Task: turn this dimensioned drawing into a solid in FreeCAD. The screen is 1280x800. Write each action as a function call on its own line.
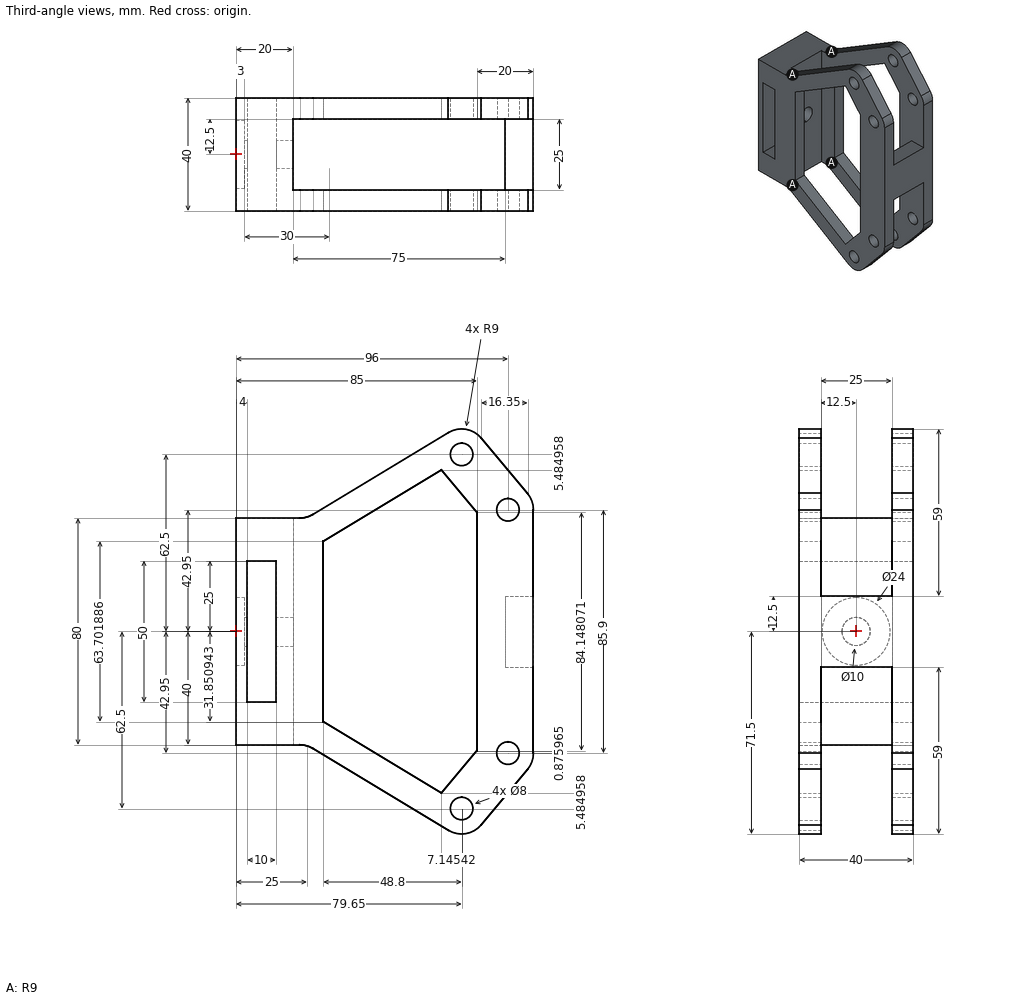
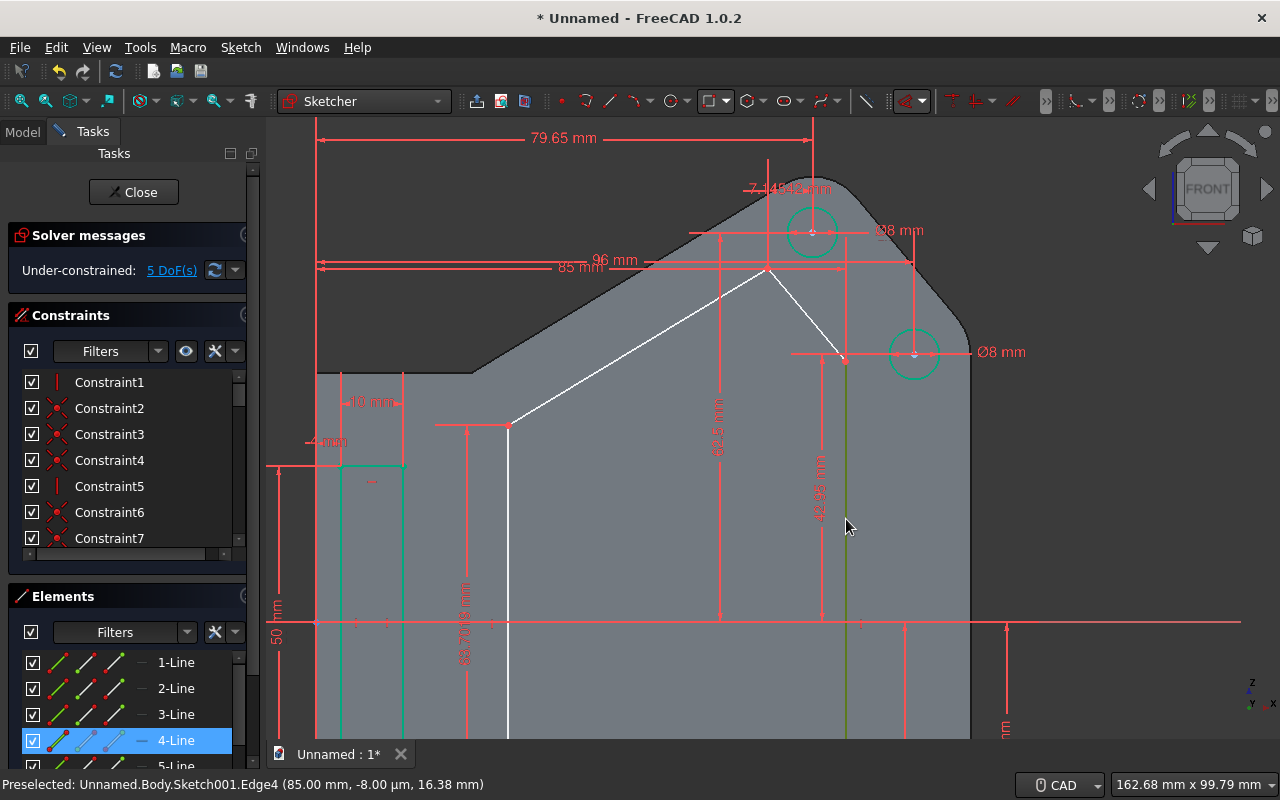
key(i)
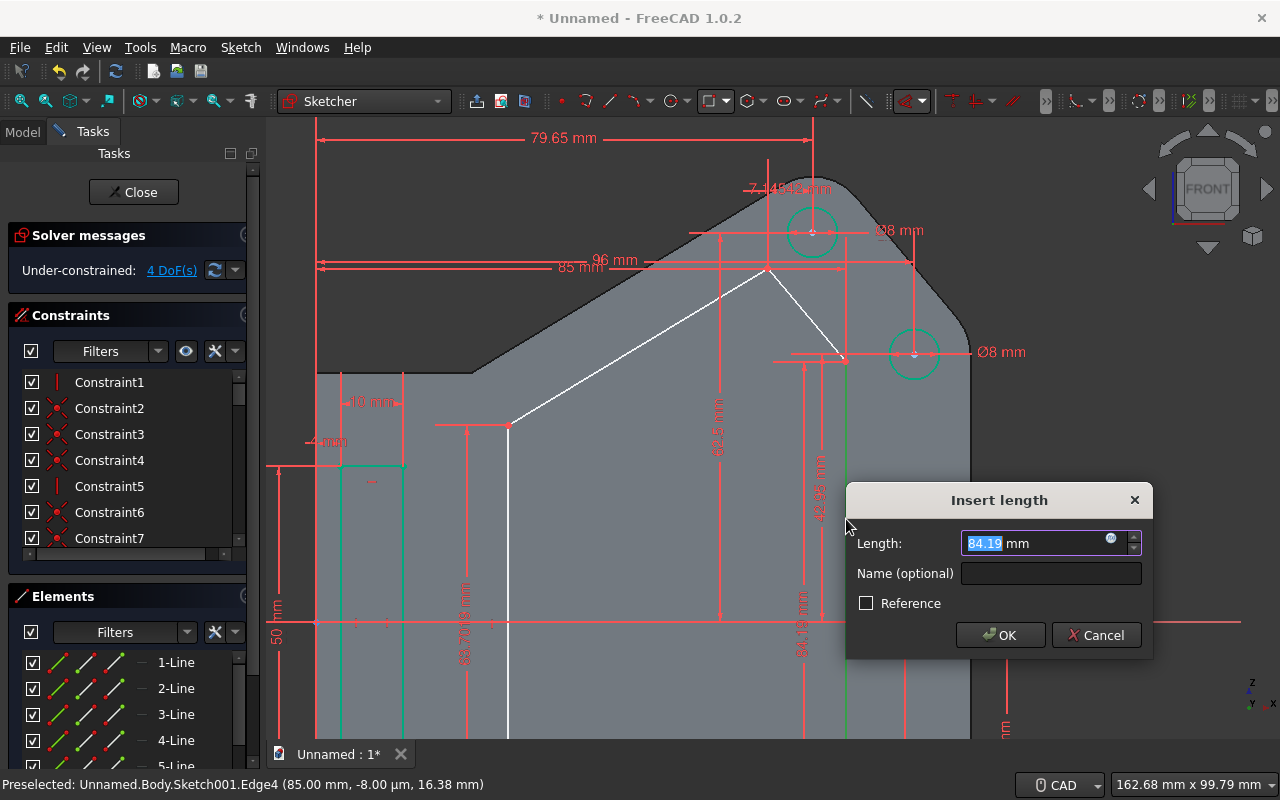
text(84.148071)
key(Return)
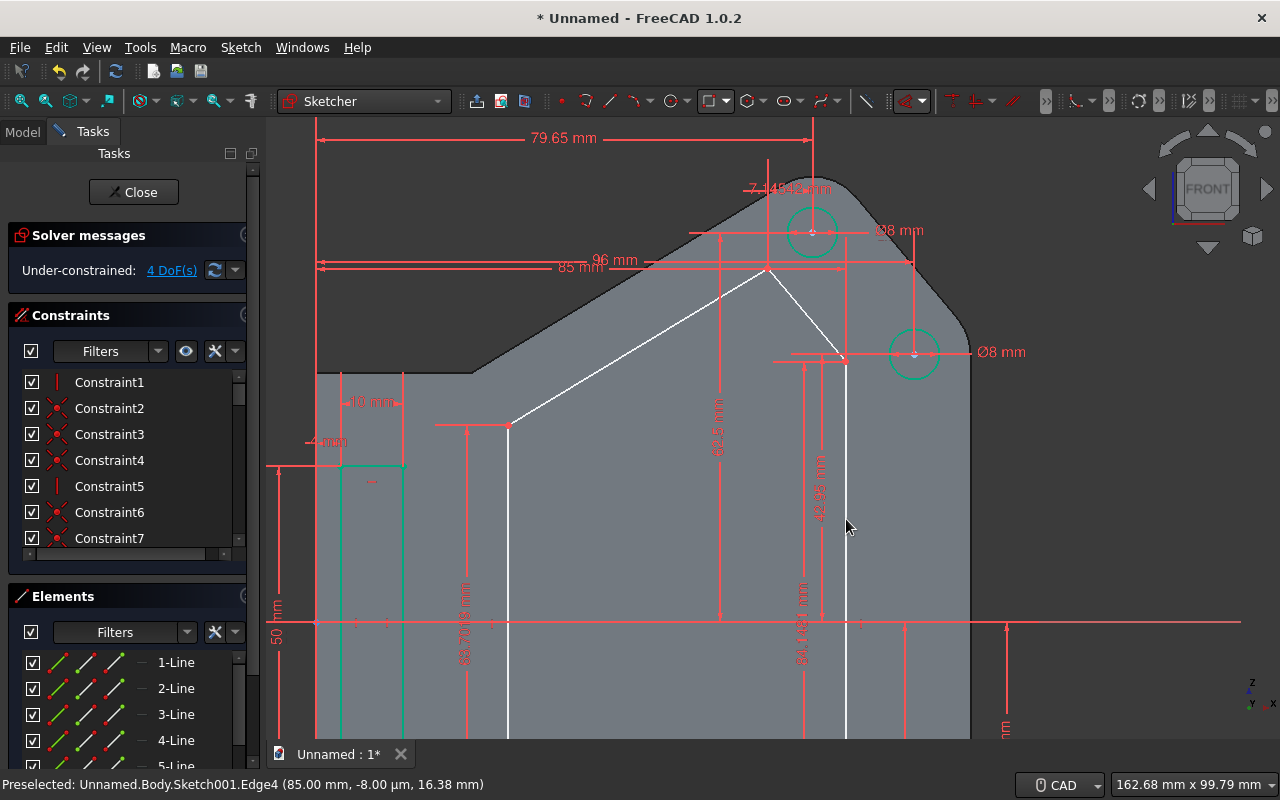
scroll(767, 270, down, 4)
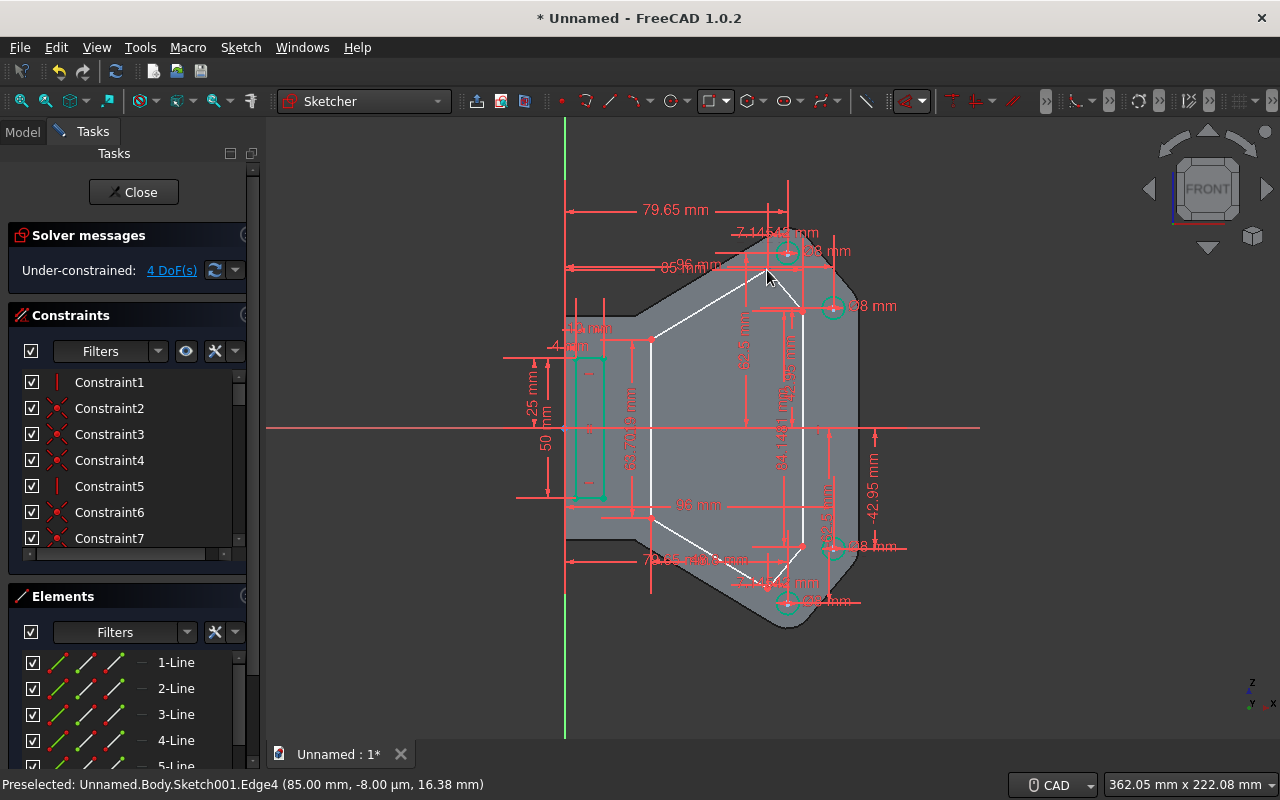
scroll(768, 589, up, 5)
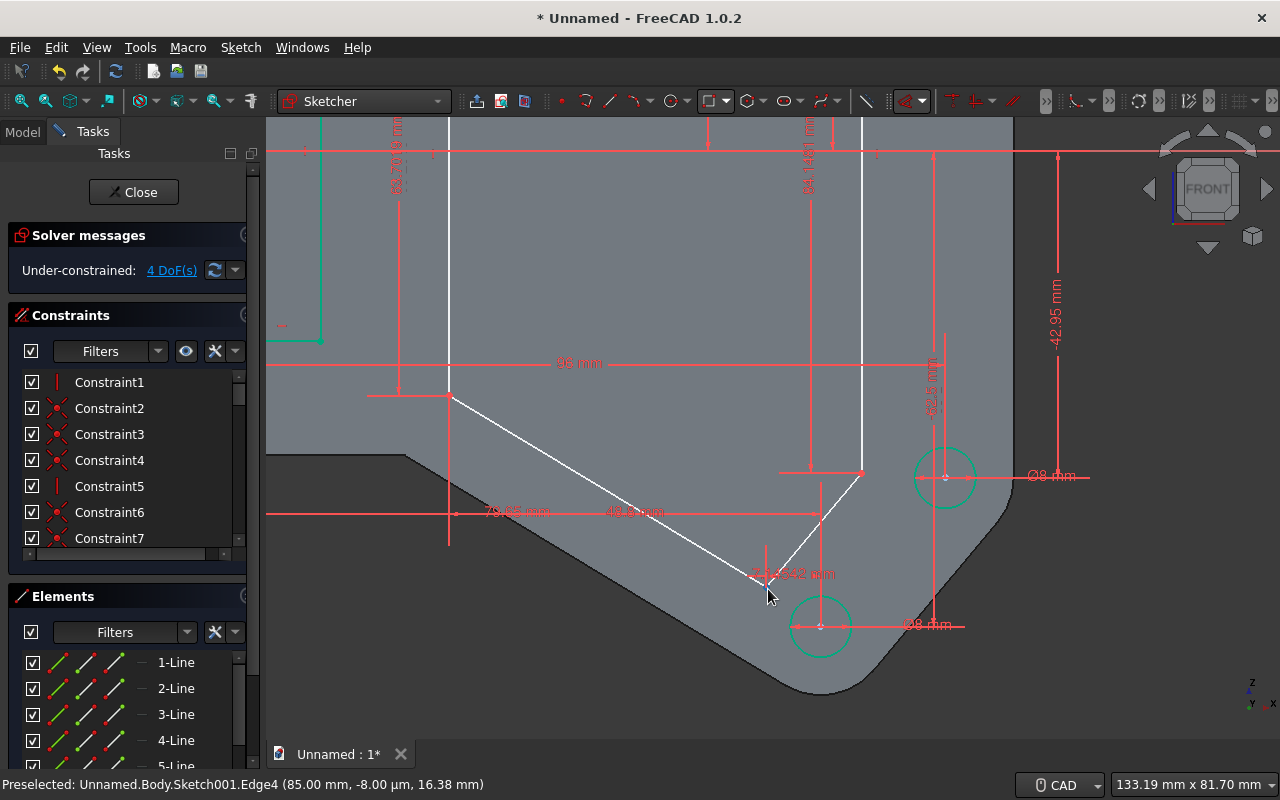
click(766, 587)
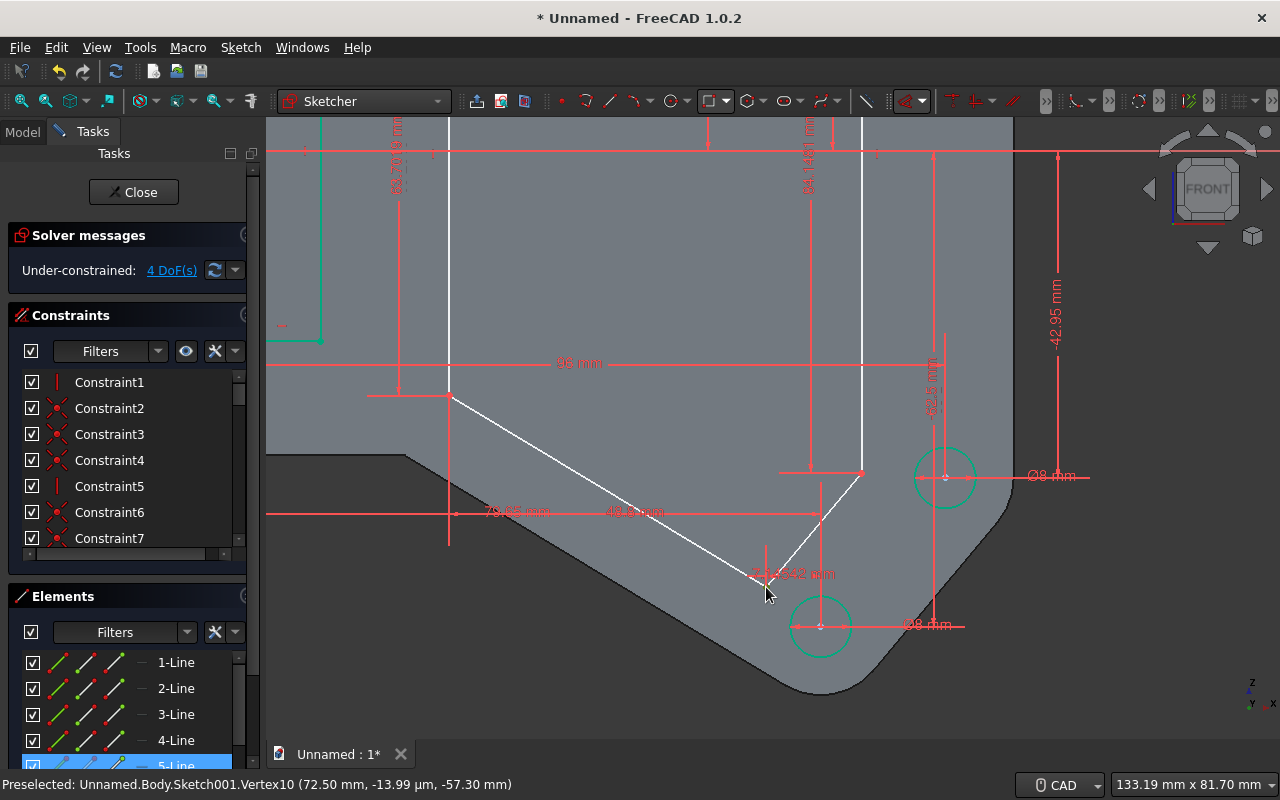
click(821, 627)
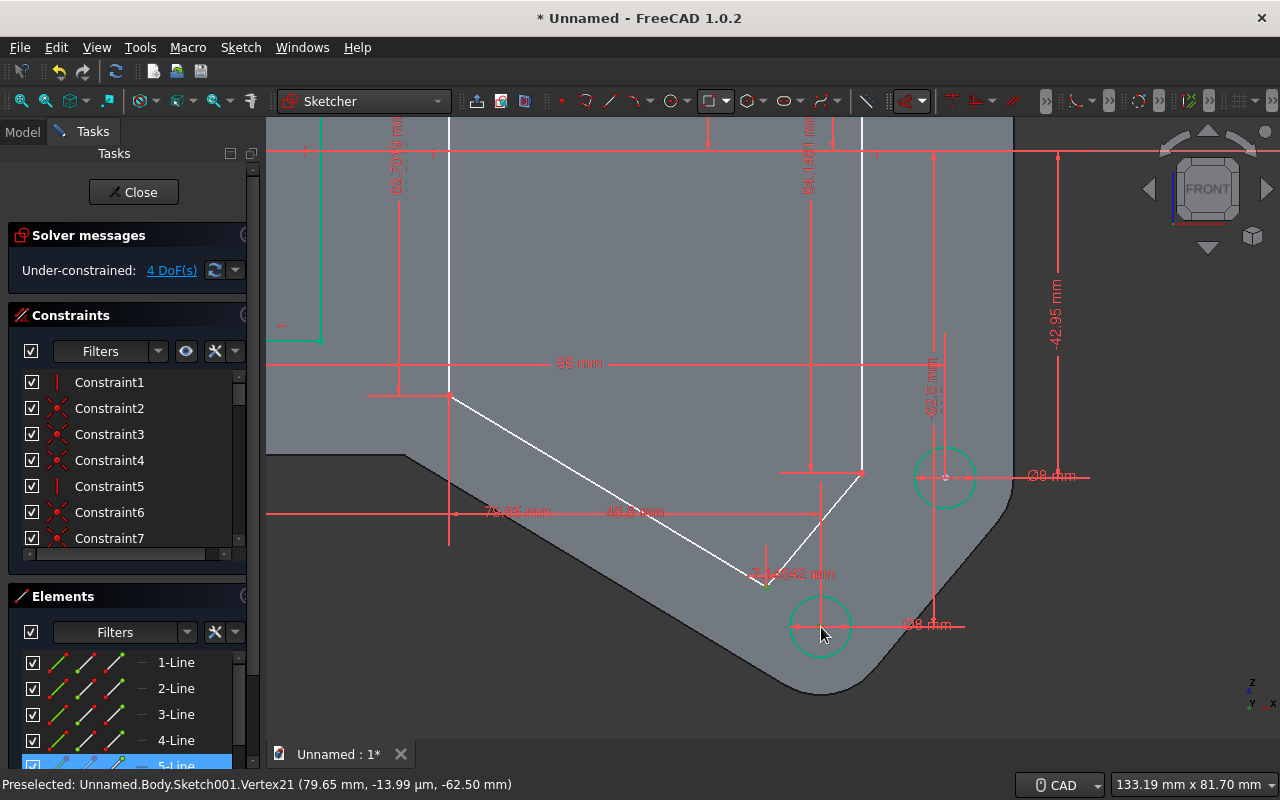
click(924, 102)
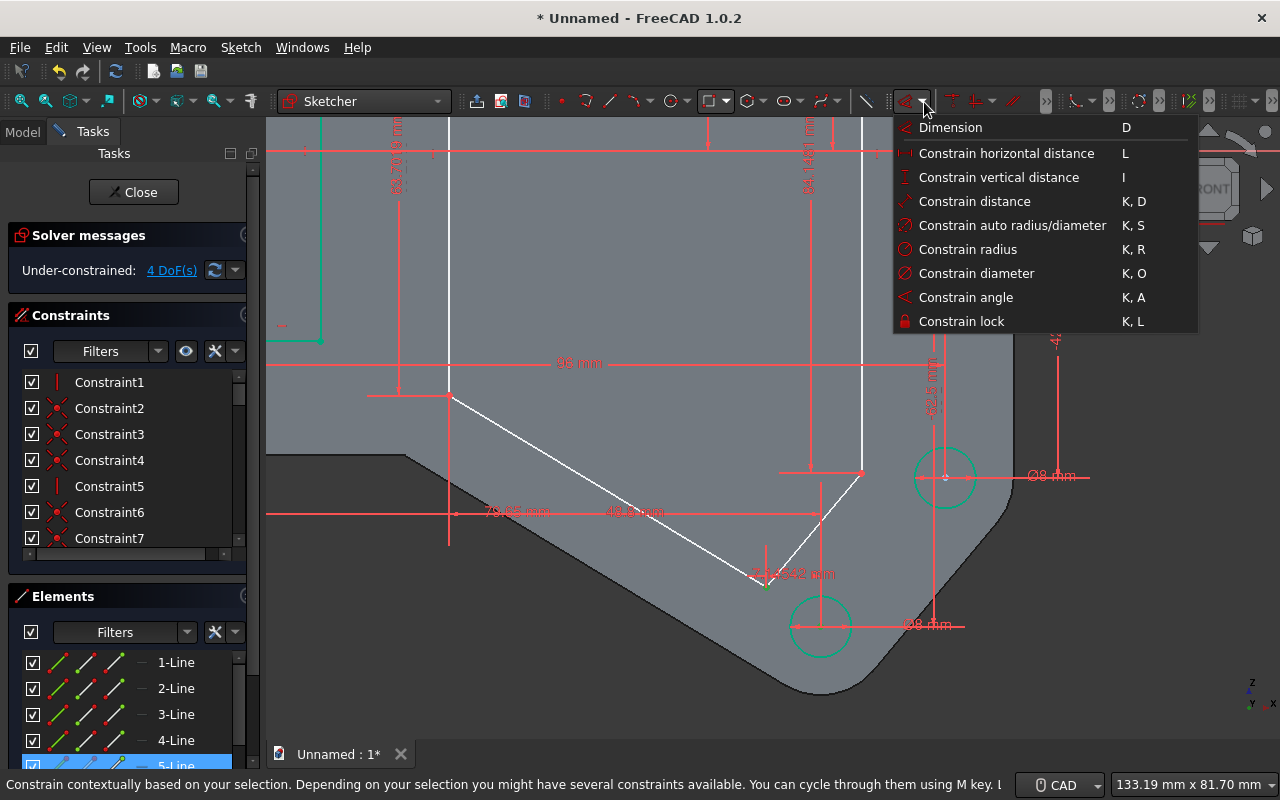
click(1046, 177)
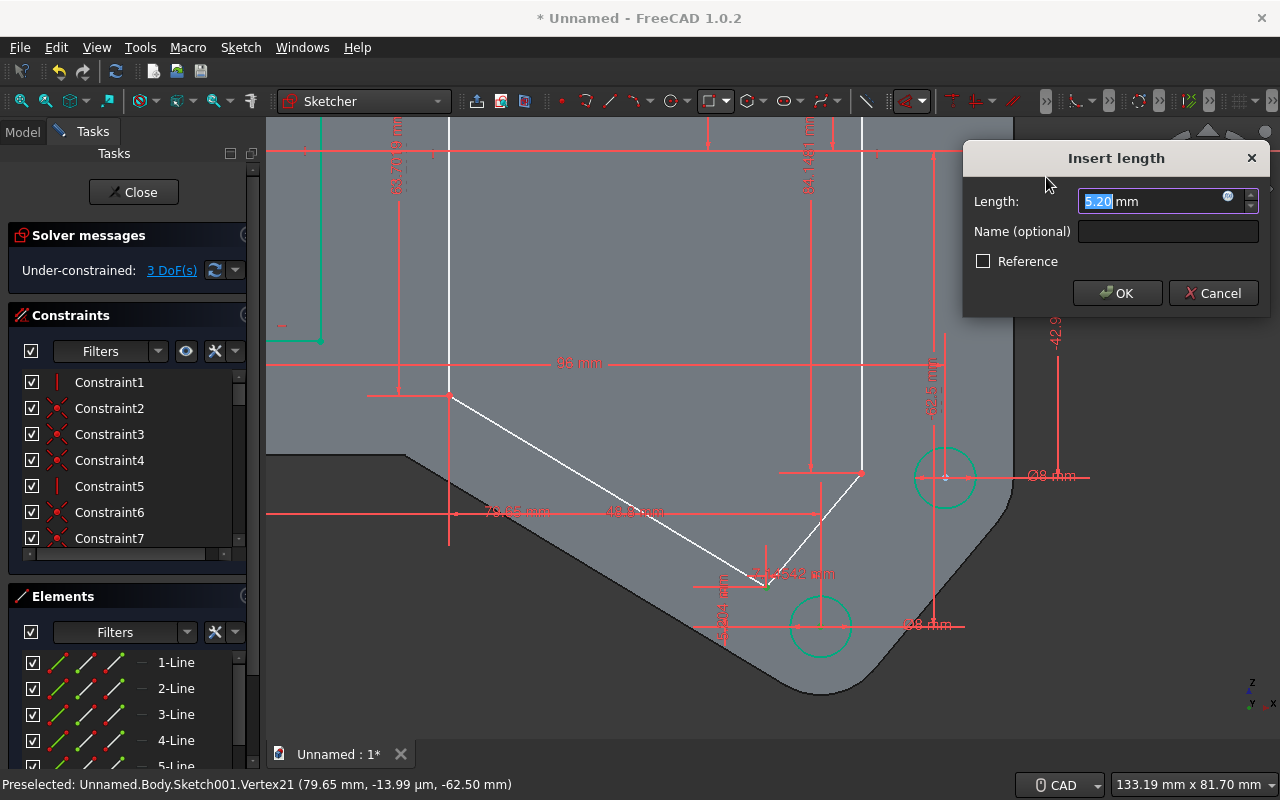
text(5.484958)
key(Return)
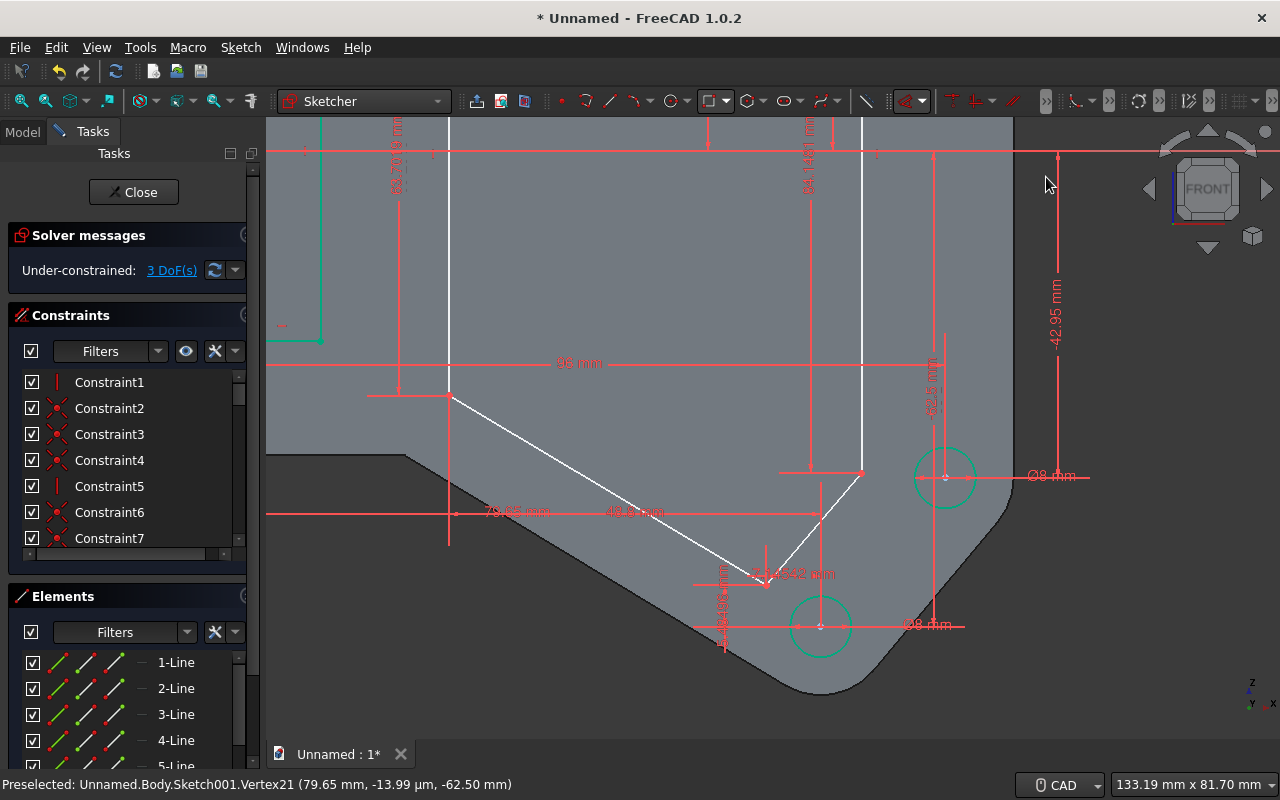
scroll(862, 473, up, 9)